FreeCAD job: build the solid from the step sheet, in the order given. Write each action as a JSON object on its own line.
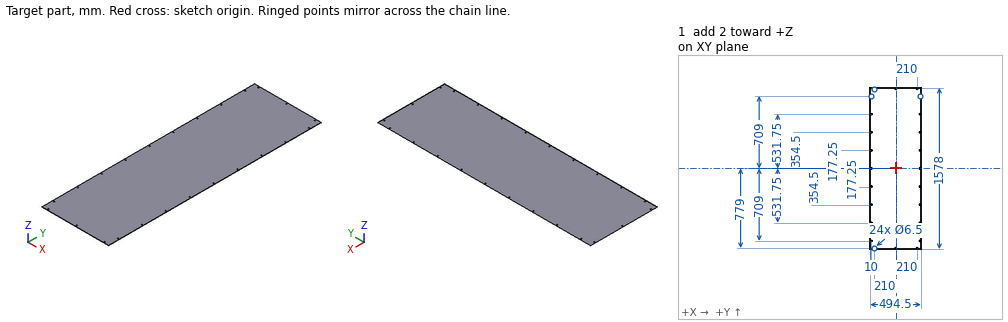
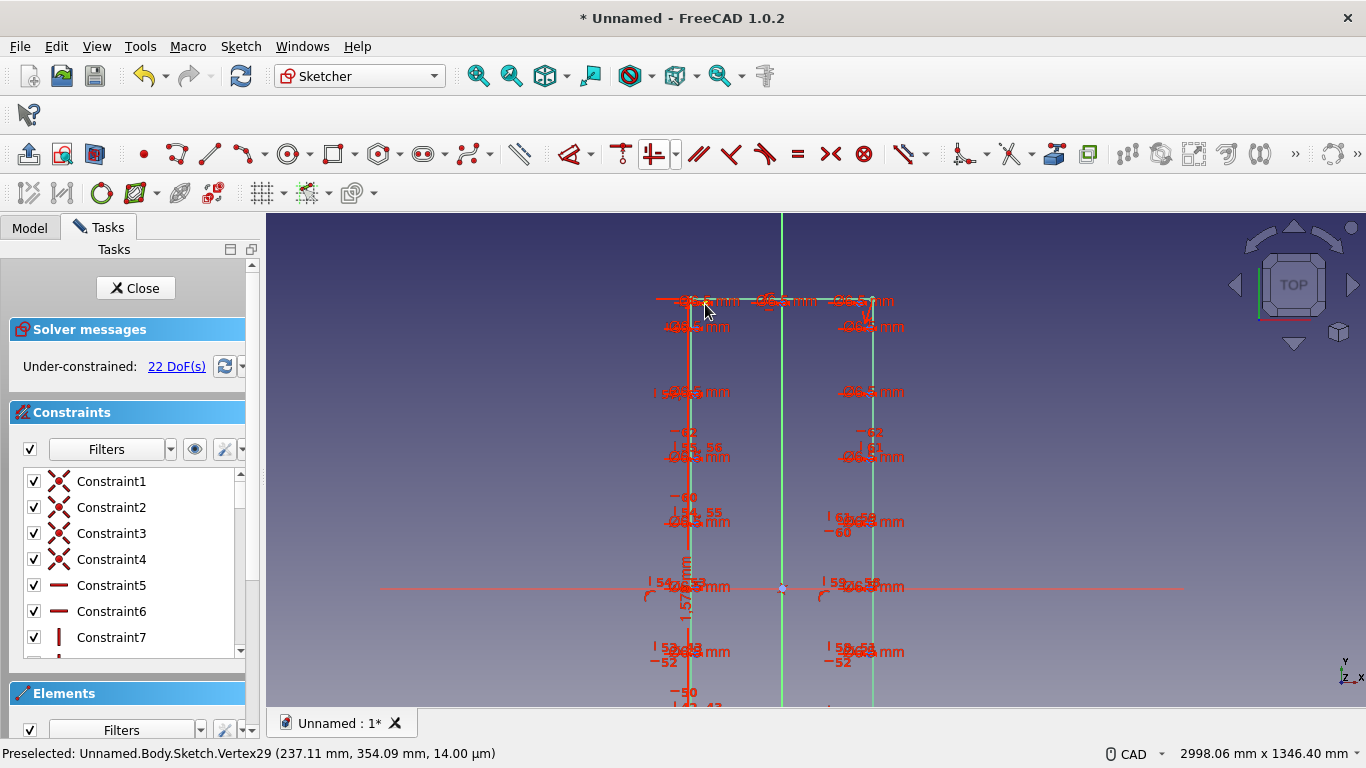
{"action": "left_click", "coordinate": [705, 303]}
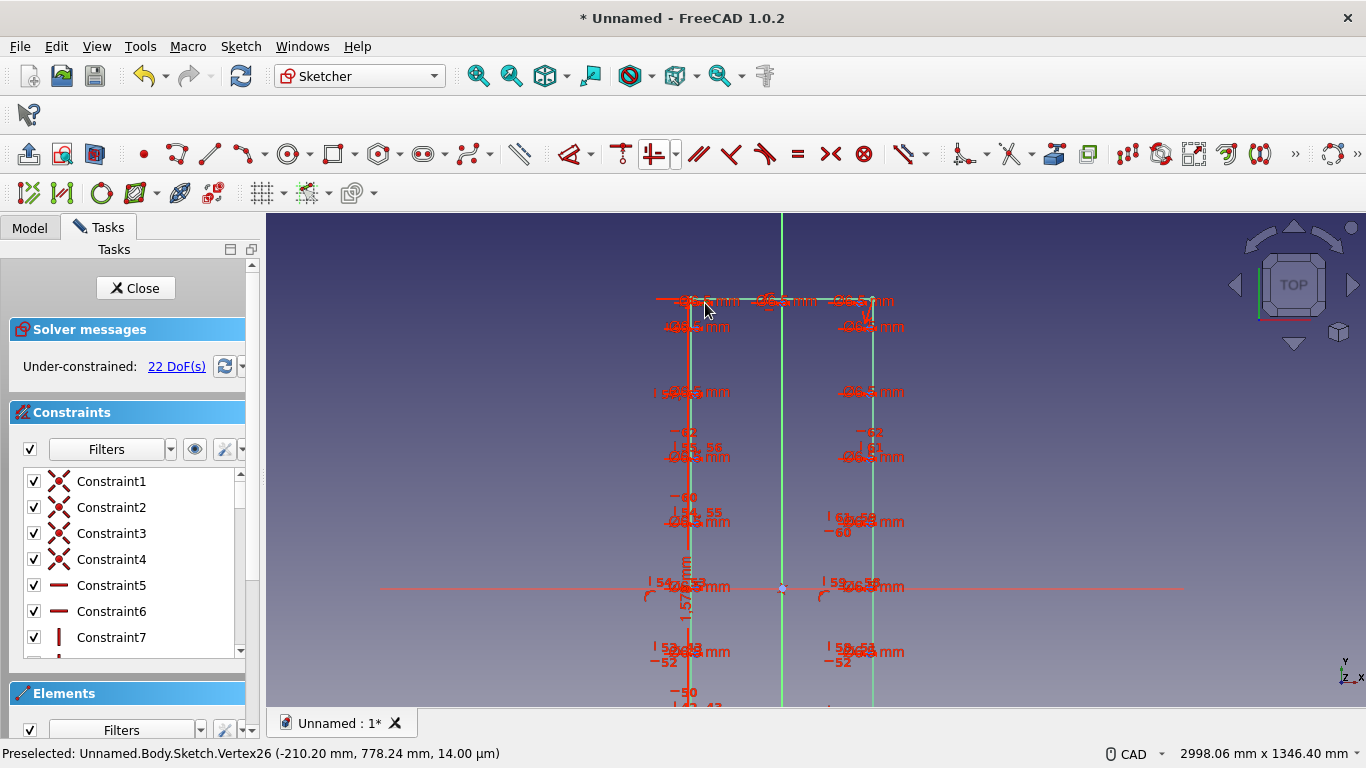
{"action": "left_click", "coordinate": [782, 303]}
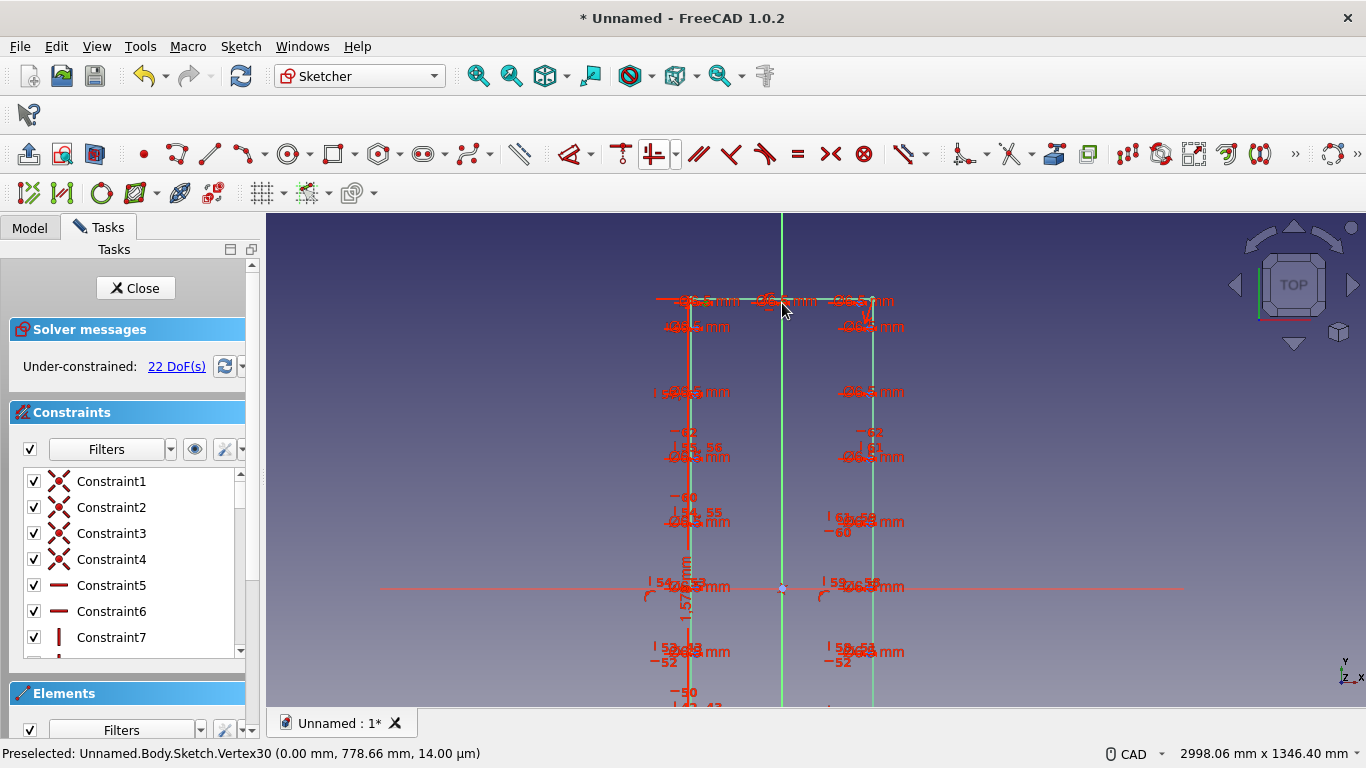
{"action": "key", "text": "h"}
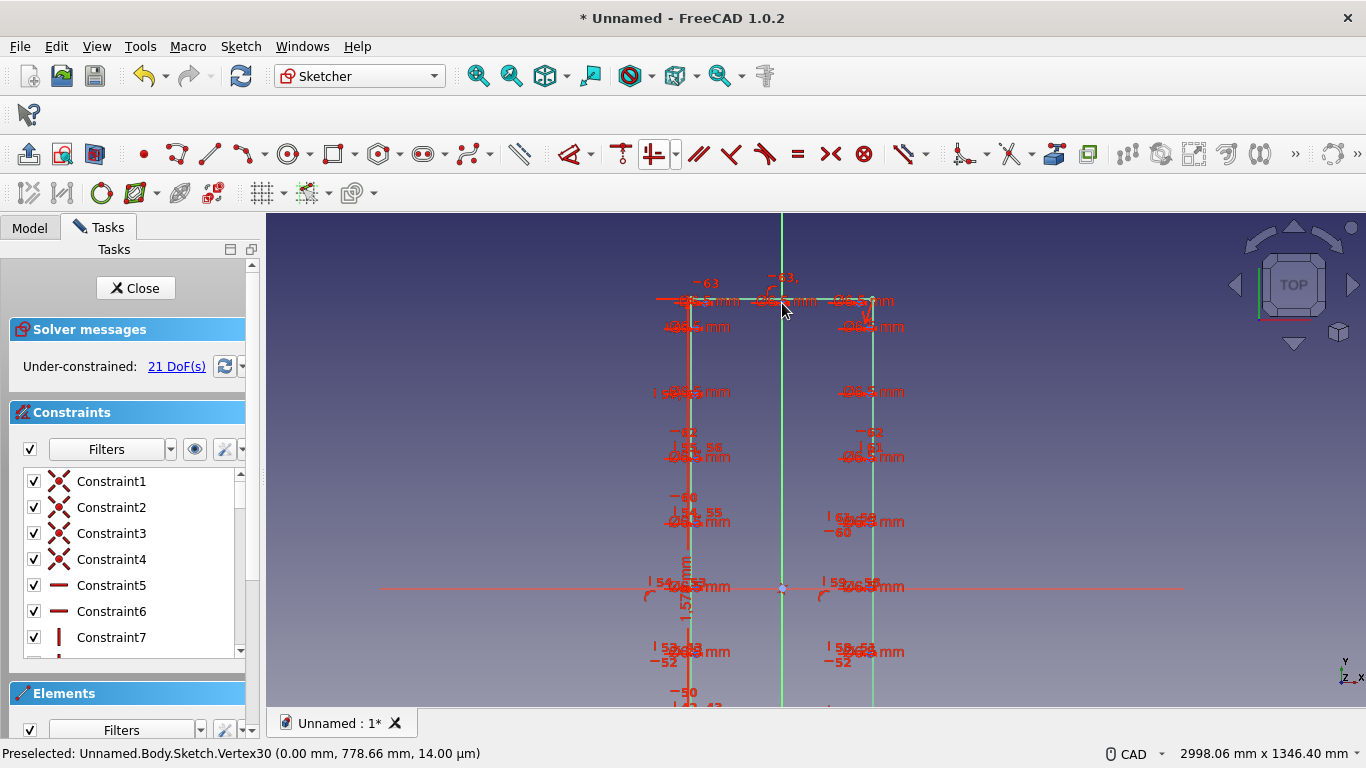
{"action": "left_click", "coordinate": [869, 459]}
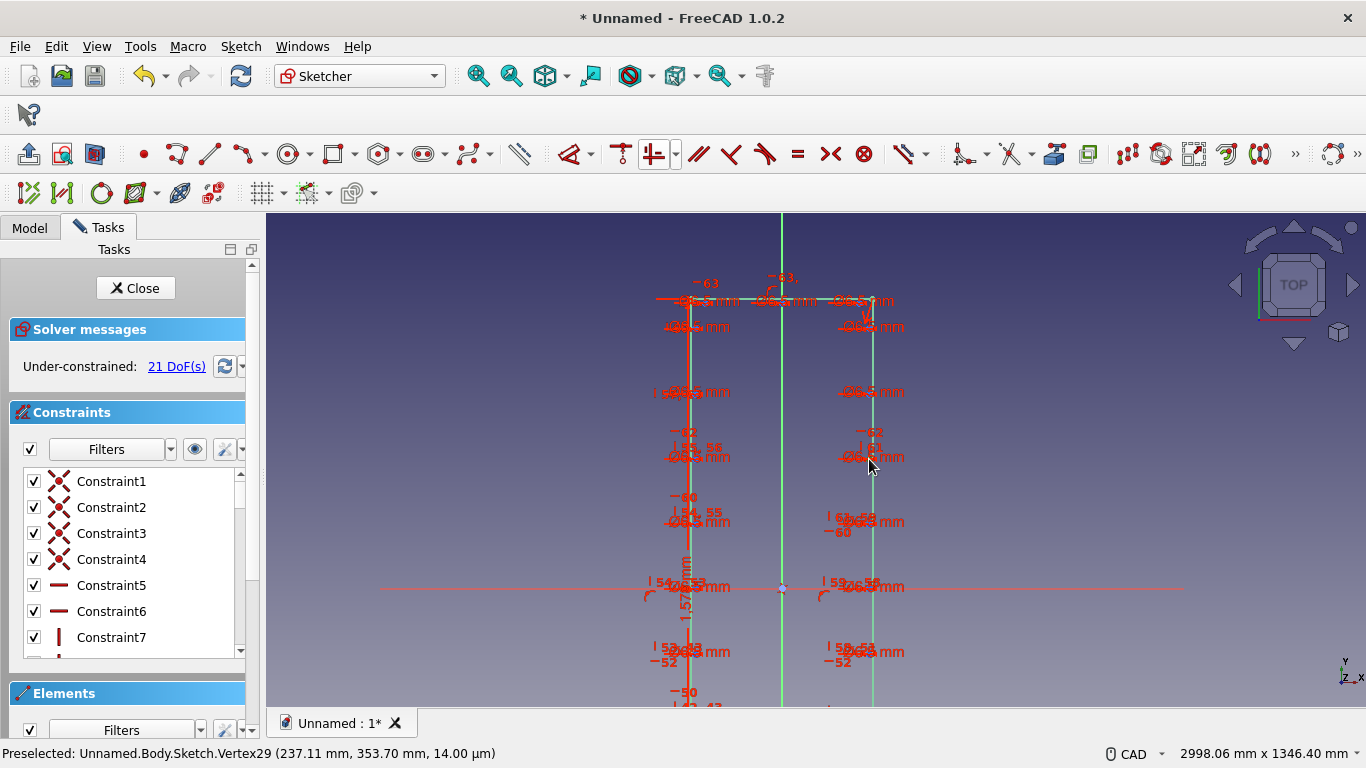
{"action": "left_click", "coordinate": [869, 394]}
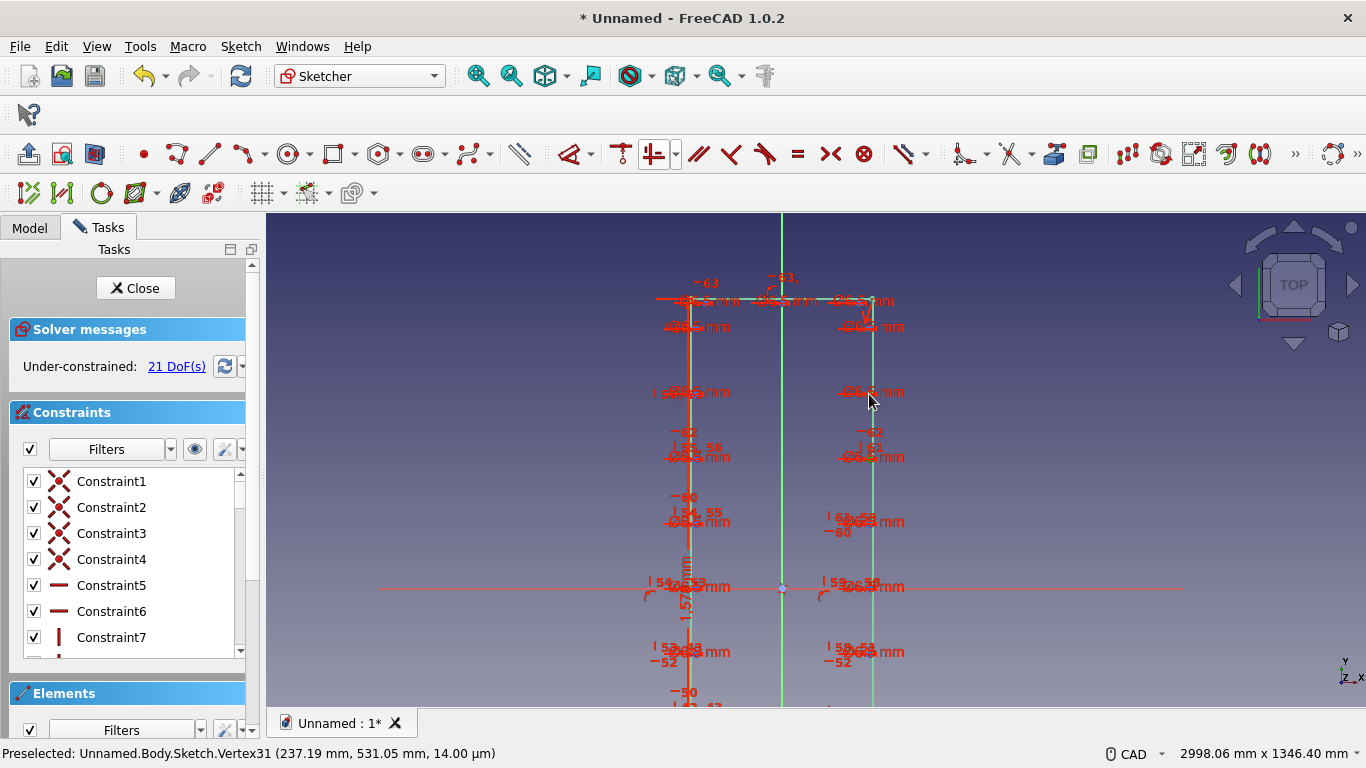
{"action": "key", "text": "v"}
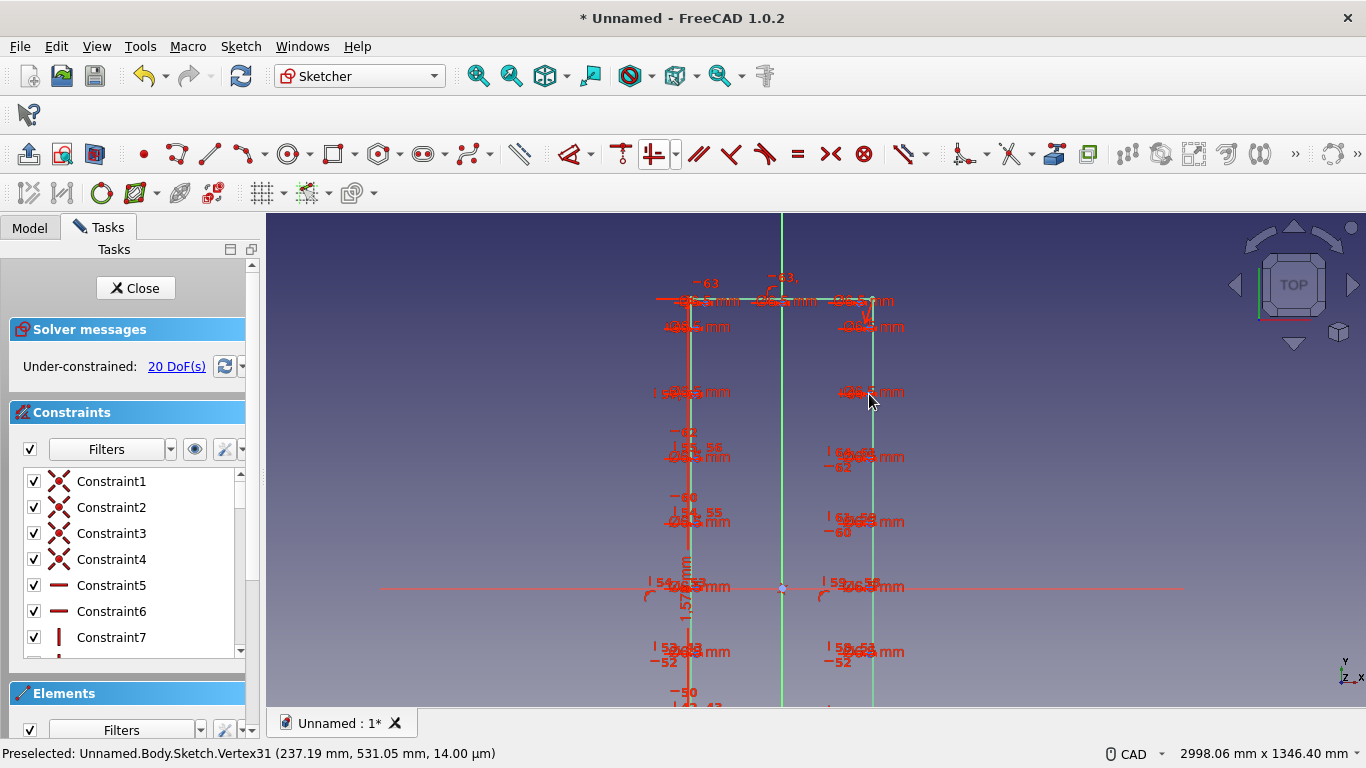
{"action": "left_click", "coordinate": [695, 394]}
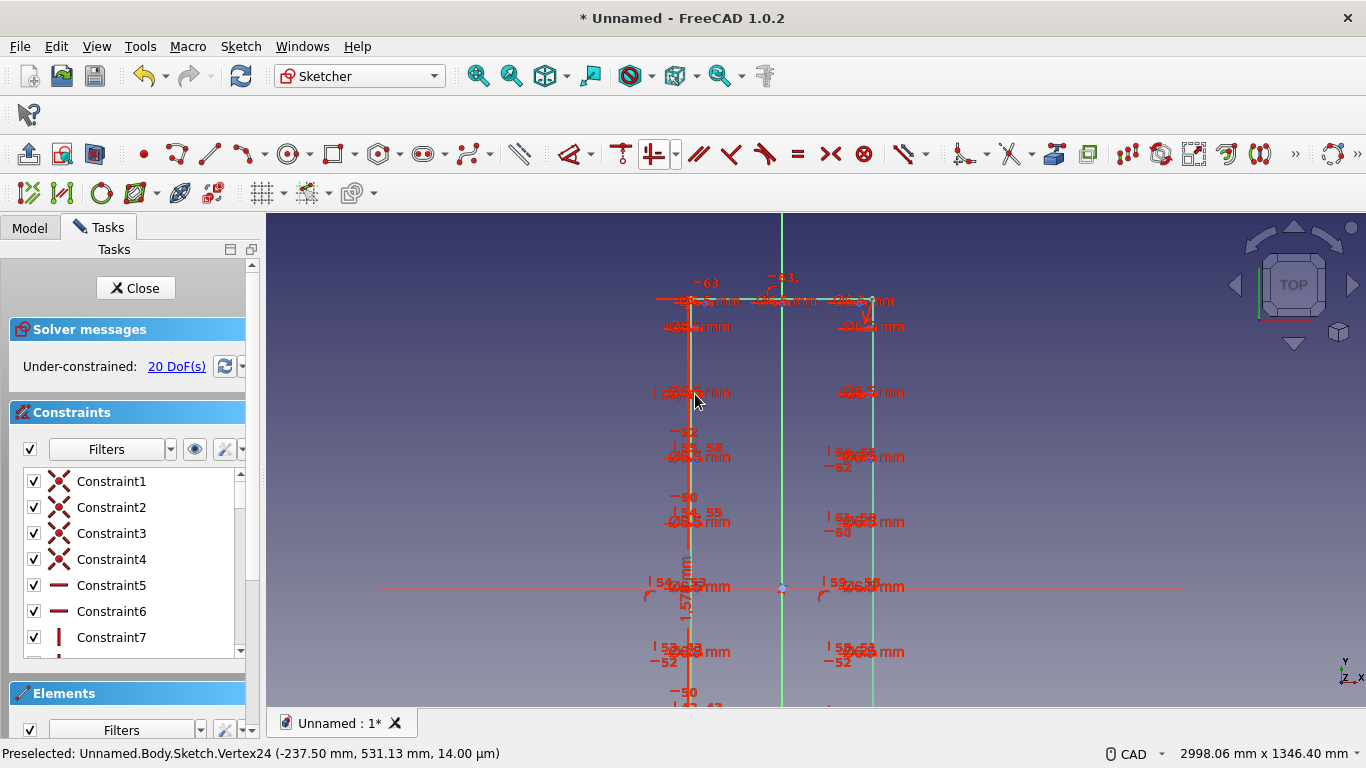
{"action": "left_click", "coordinate": [869, 394]}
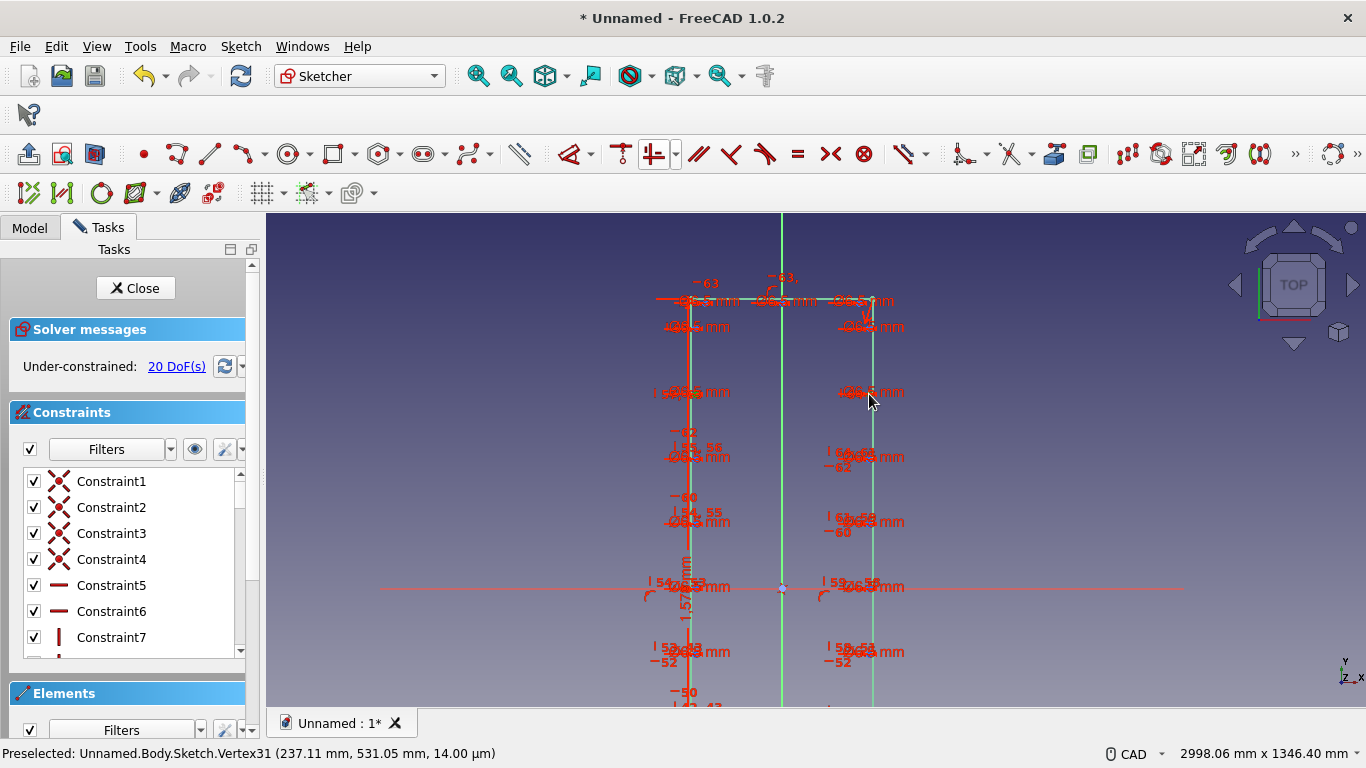
{"action": "key", "text": "h"}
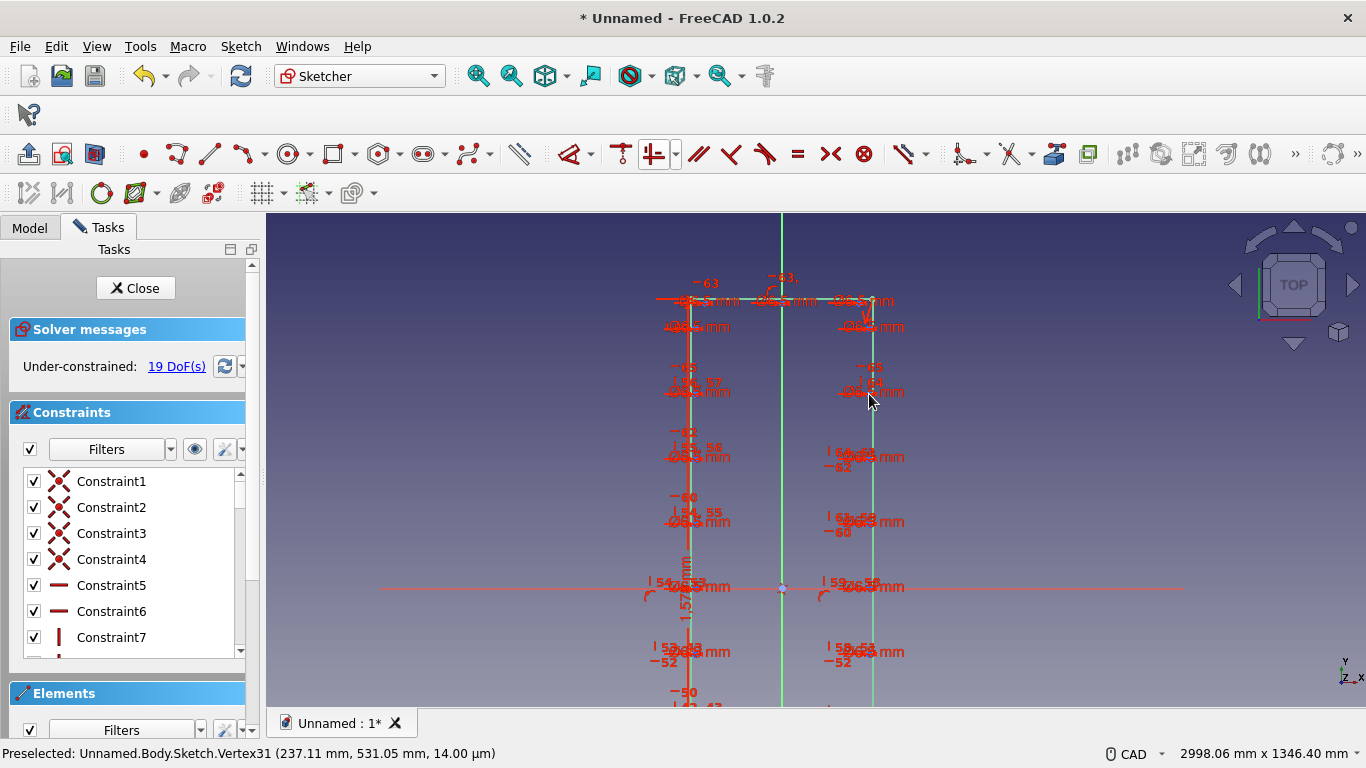
{"action": "left_click", "coordinate": [782, 303]}